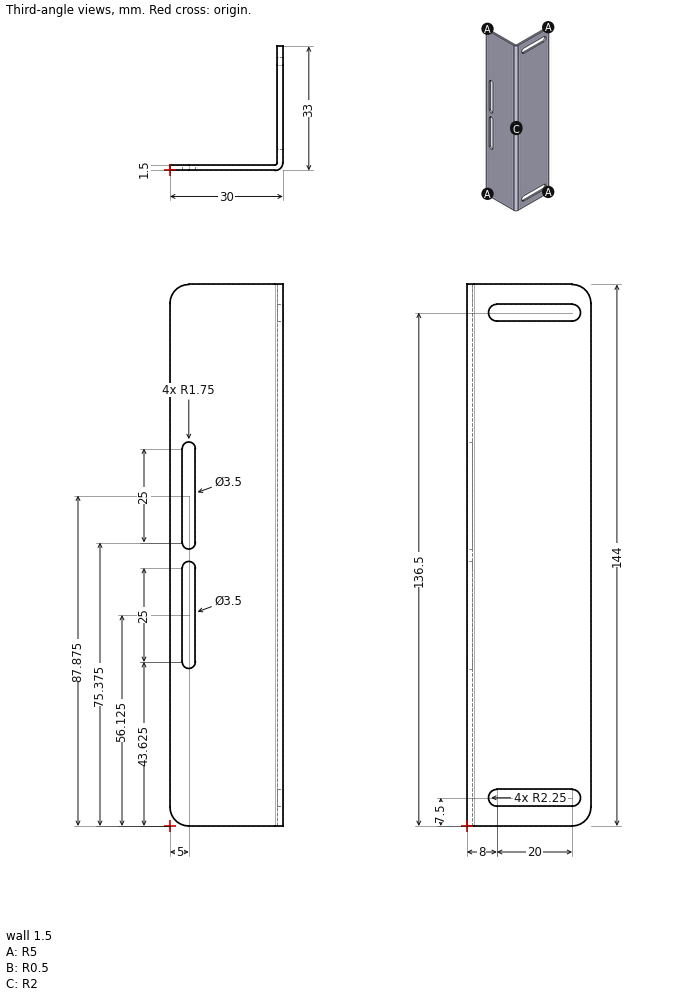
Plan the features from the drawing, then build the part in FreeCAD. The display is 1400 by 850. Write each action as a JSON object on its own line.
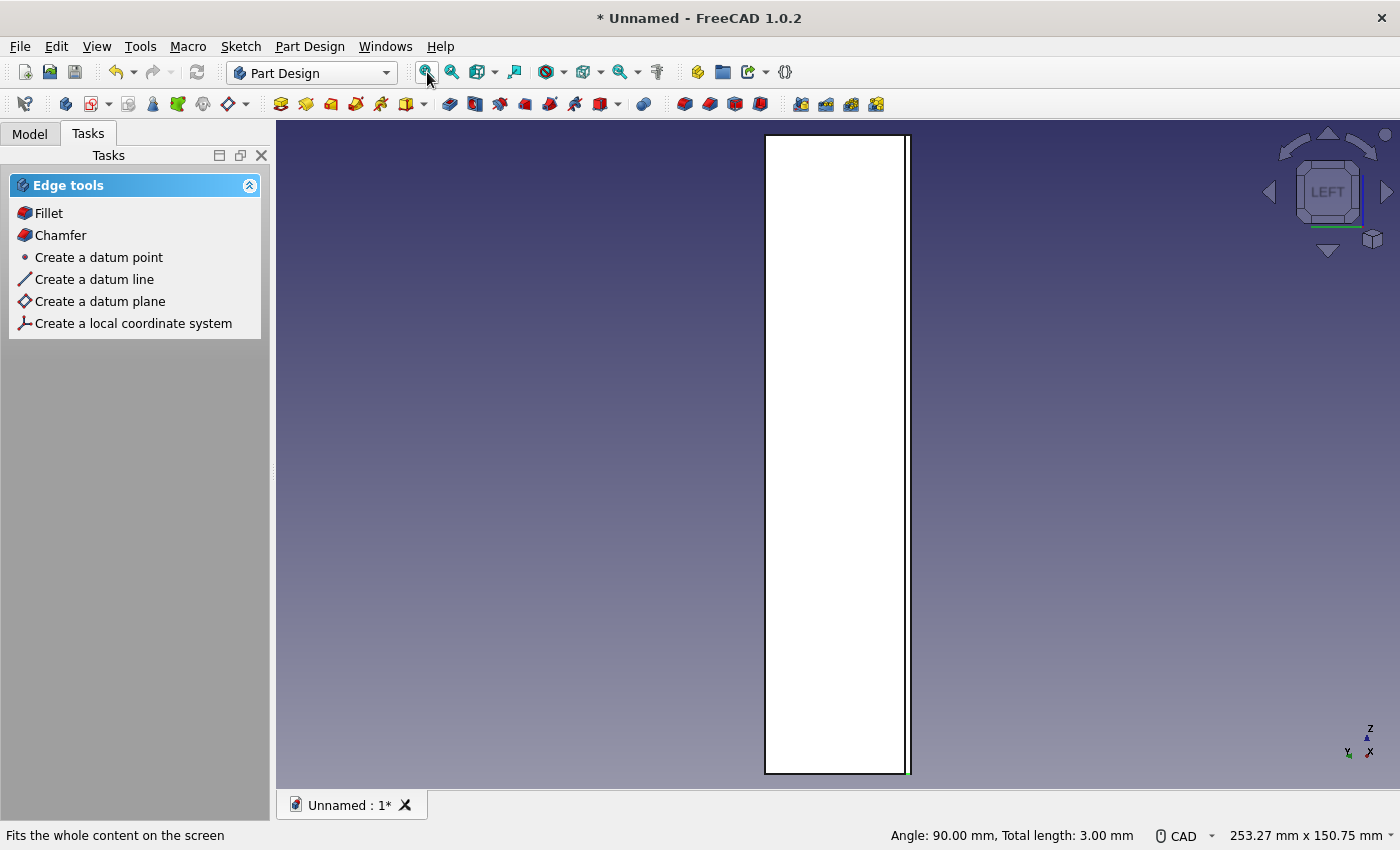
{"action": "key", "text": "v 3"}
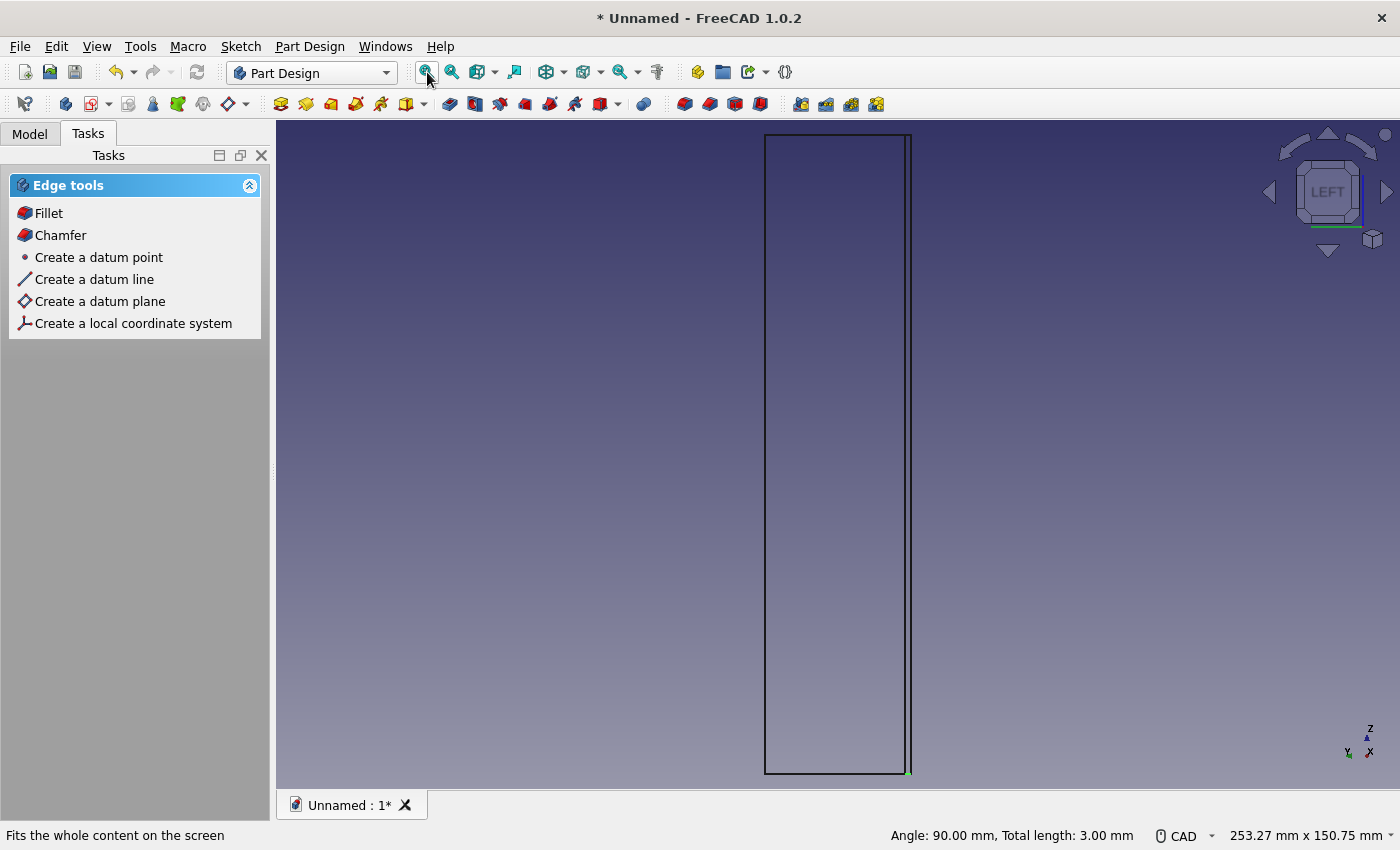
{"action": "key", "text": "0"}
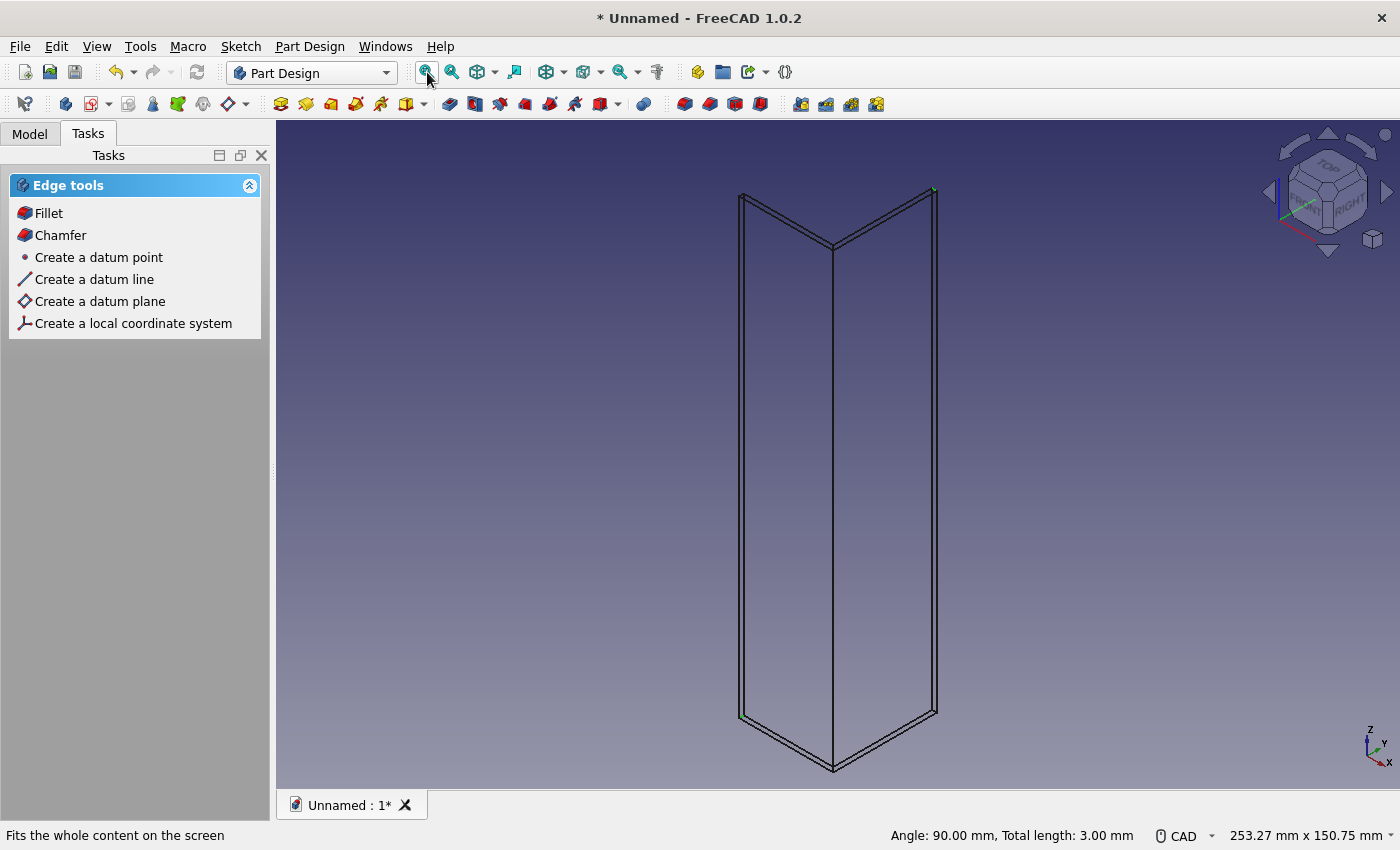
{"action": "scroll", "coordinate": [742, 194], "scroll_direction": "up", "scroll_amount": 9}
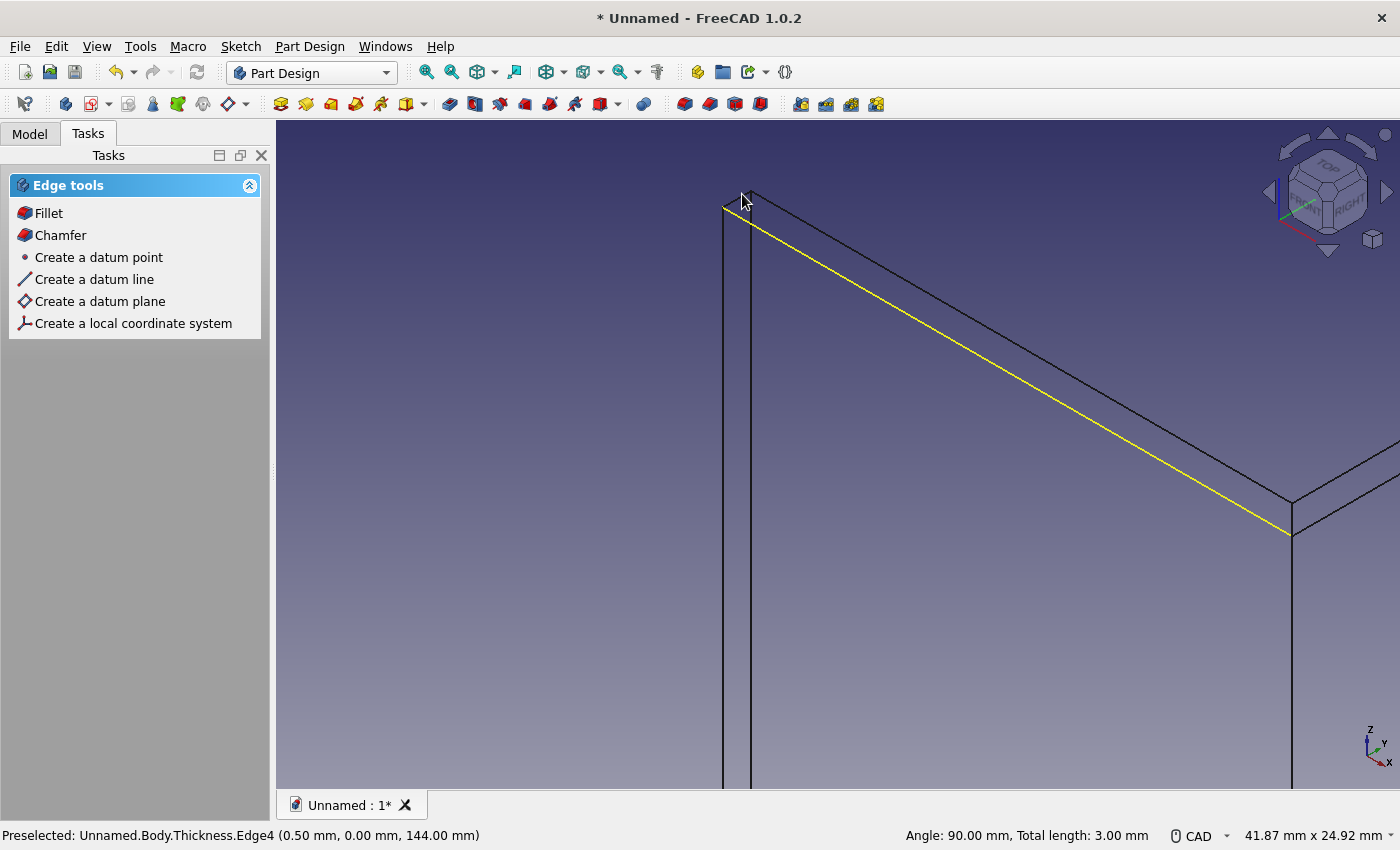
{"action": "left_click", "coordinate": [737, 198], "text": "ctrl"}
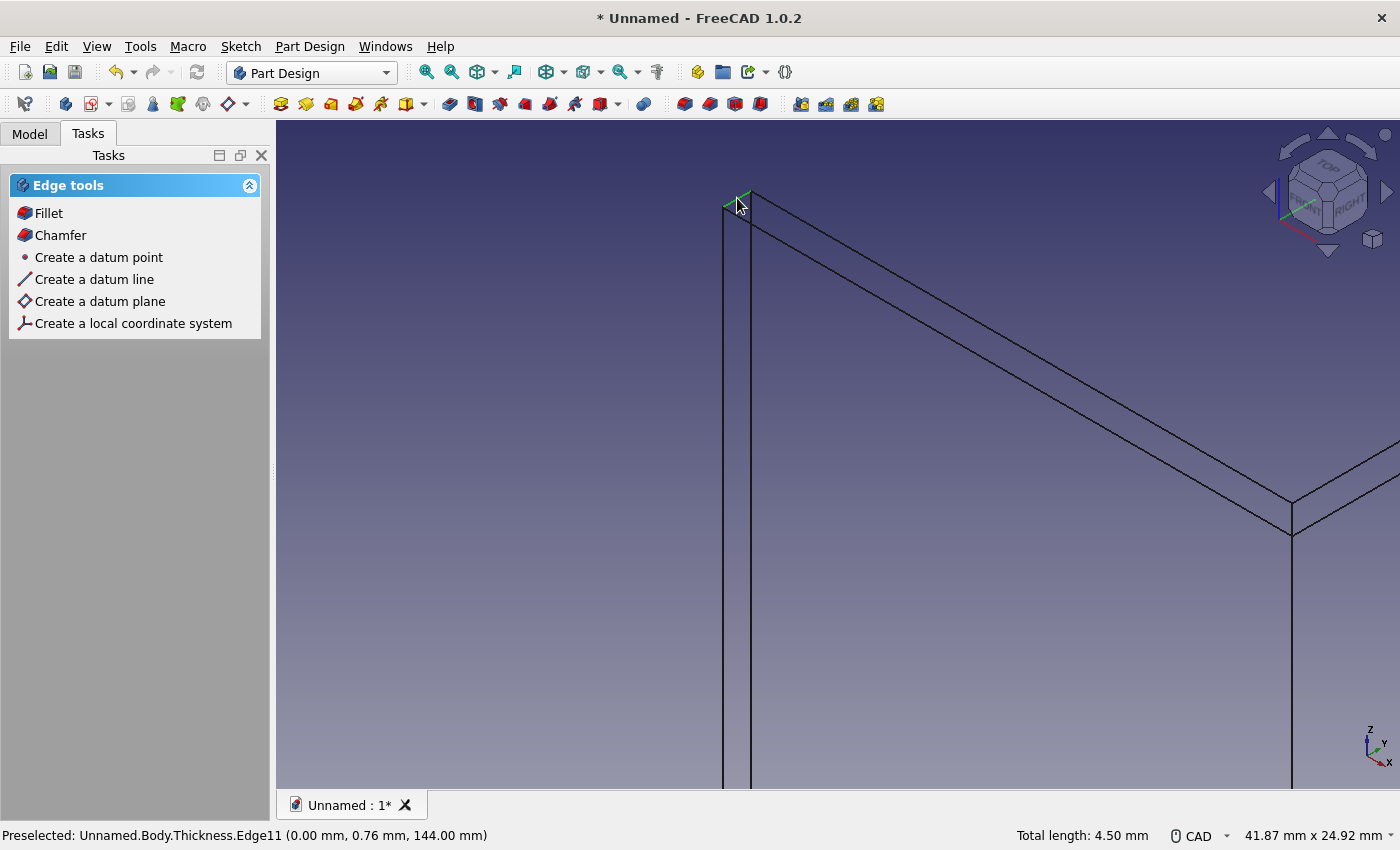
{"action": "left_click", "coordinate": [427, 72]}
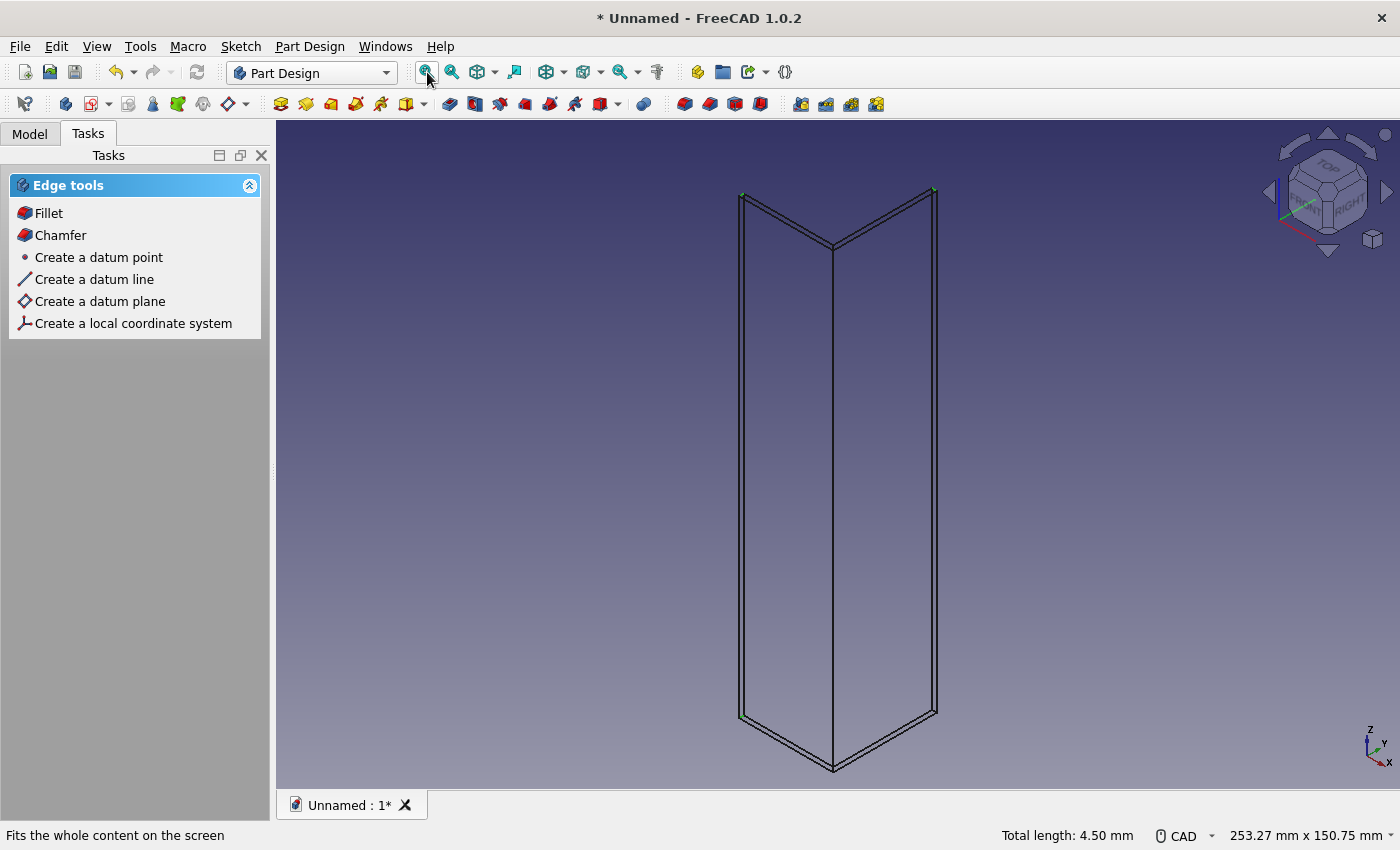
{"action": "key", "text": "2"}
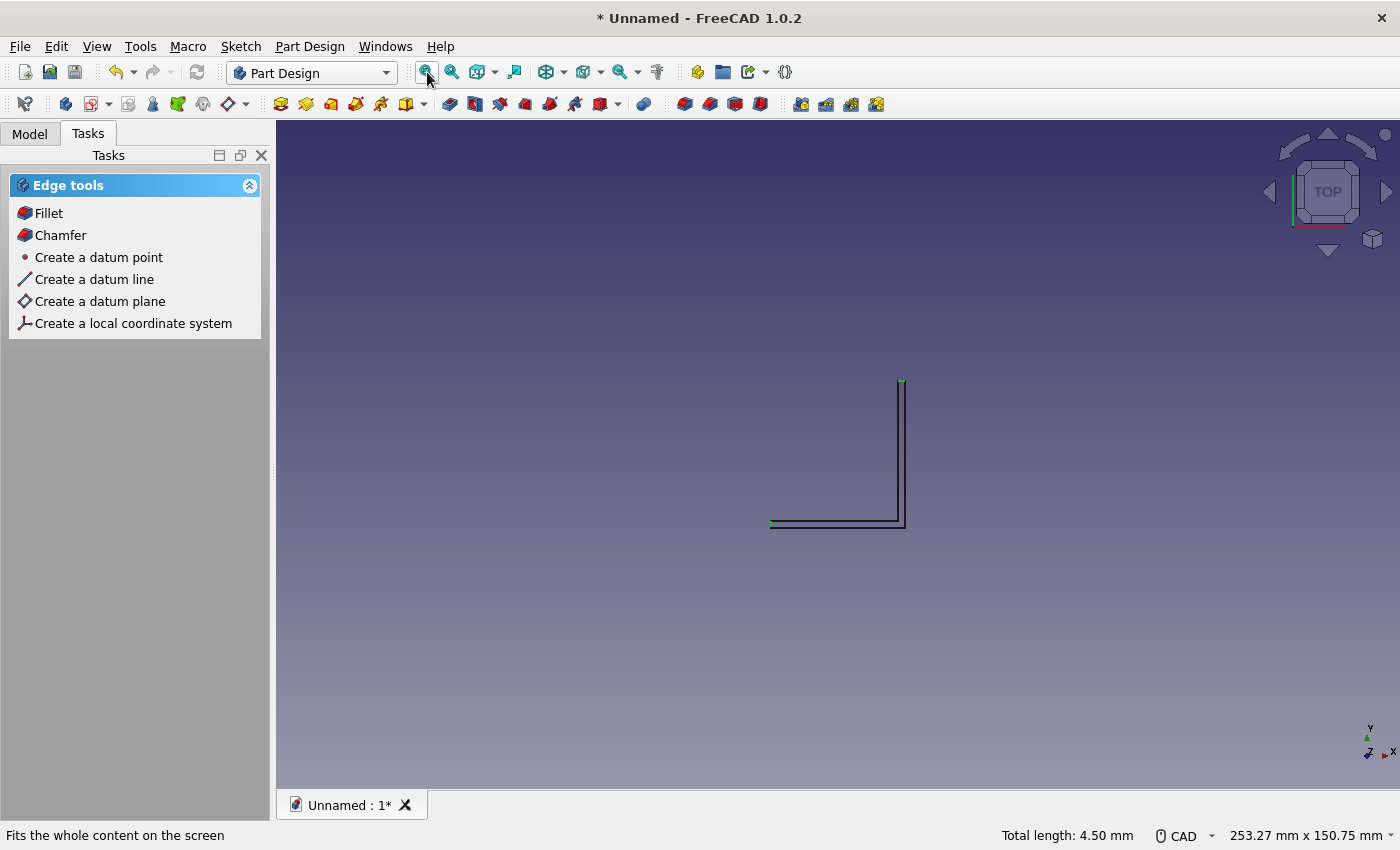
{"action": "left_click", "coordinate": [427, 72]}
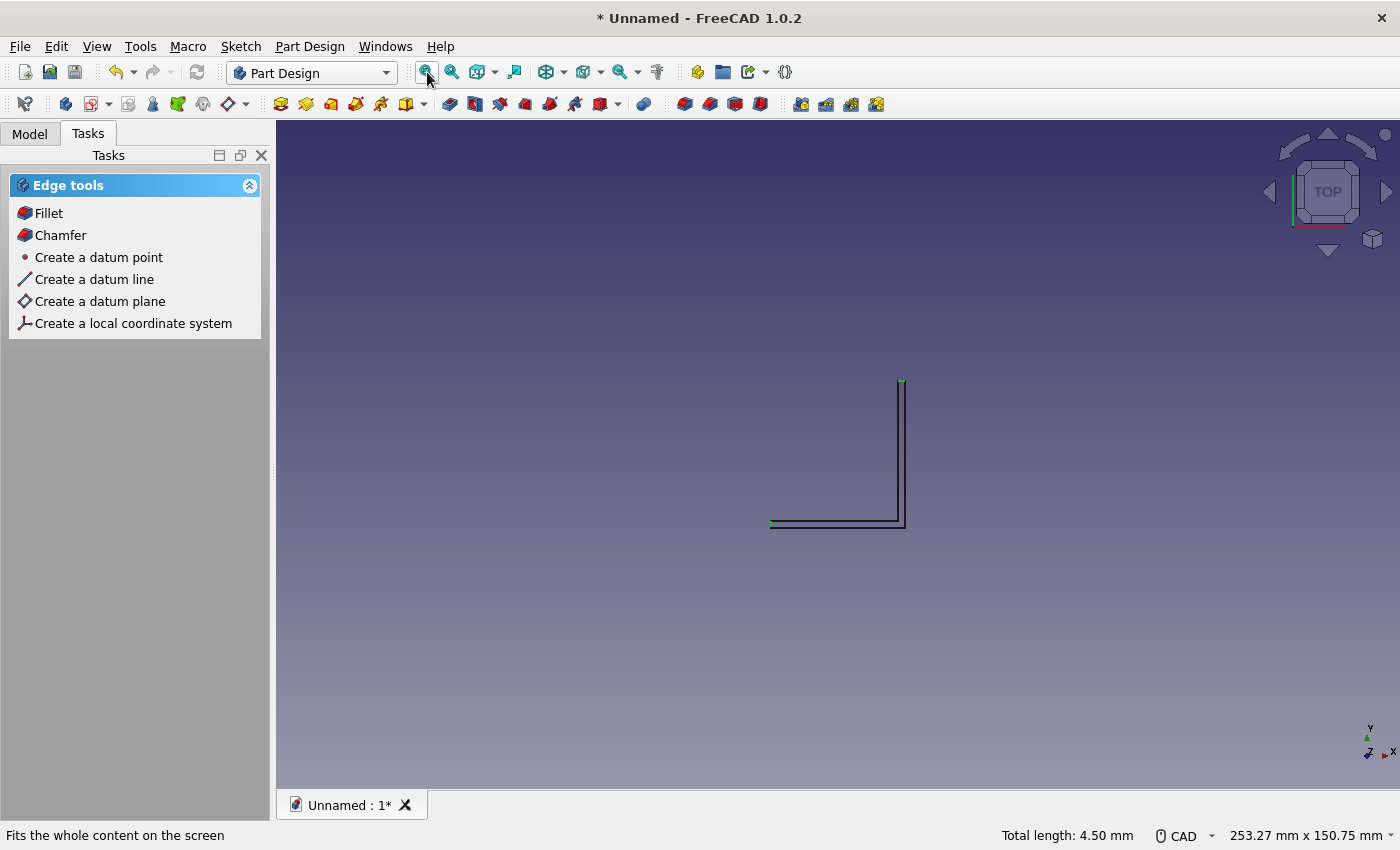
{"action": "scroll", "coordinate": [901, 380], "scroll_direction": "up", "scroll_amount": 9}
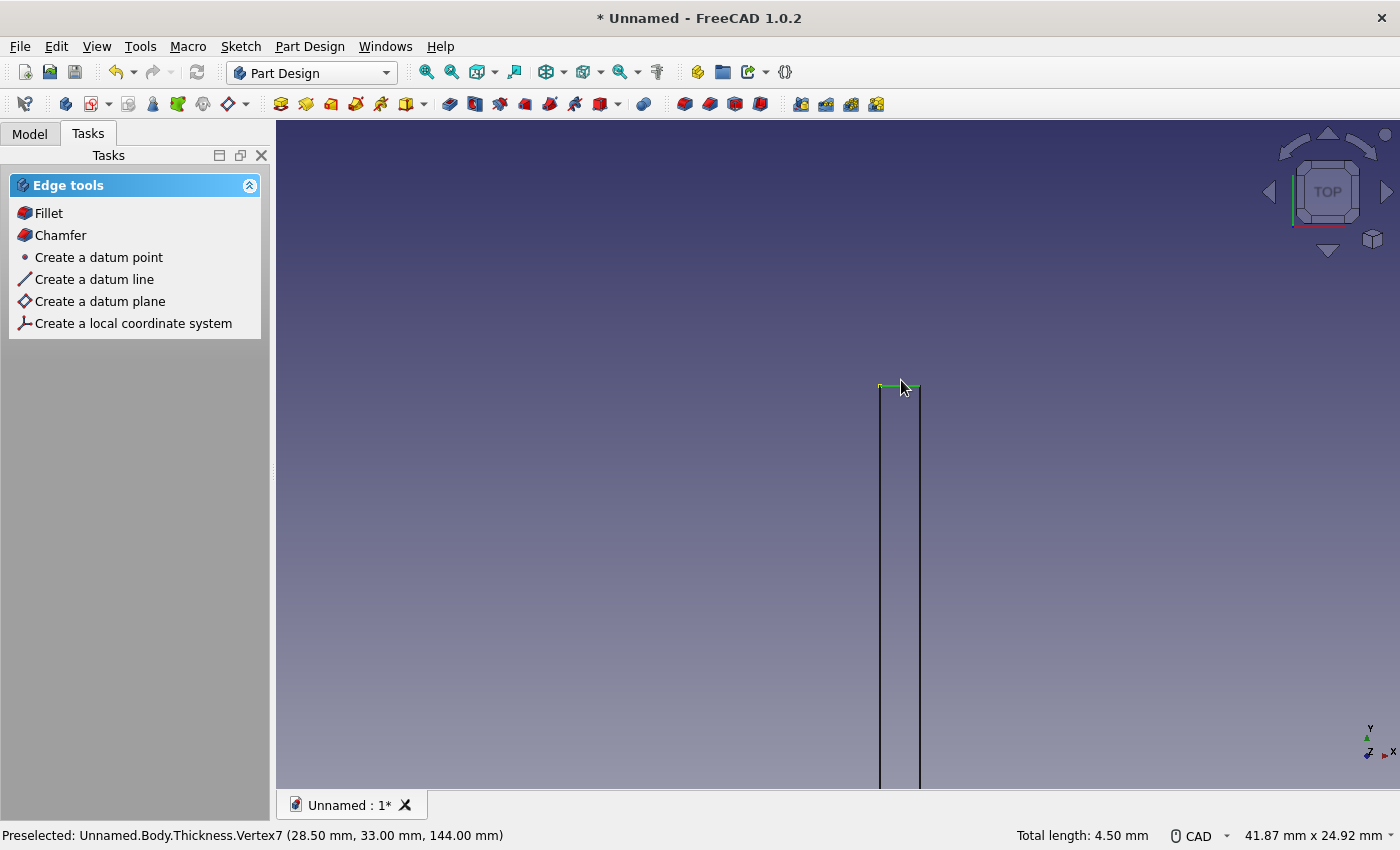
{"action": "left_click", "coordinate": [427, 72]}